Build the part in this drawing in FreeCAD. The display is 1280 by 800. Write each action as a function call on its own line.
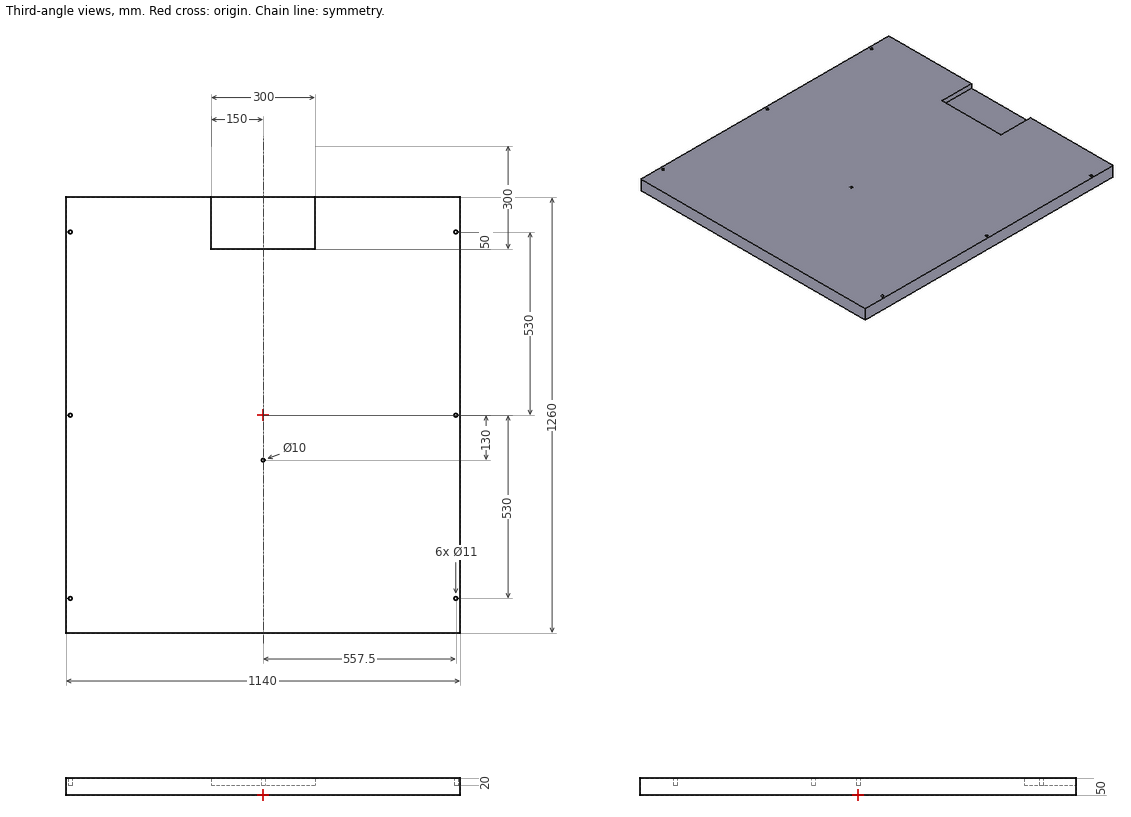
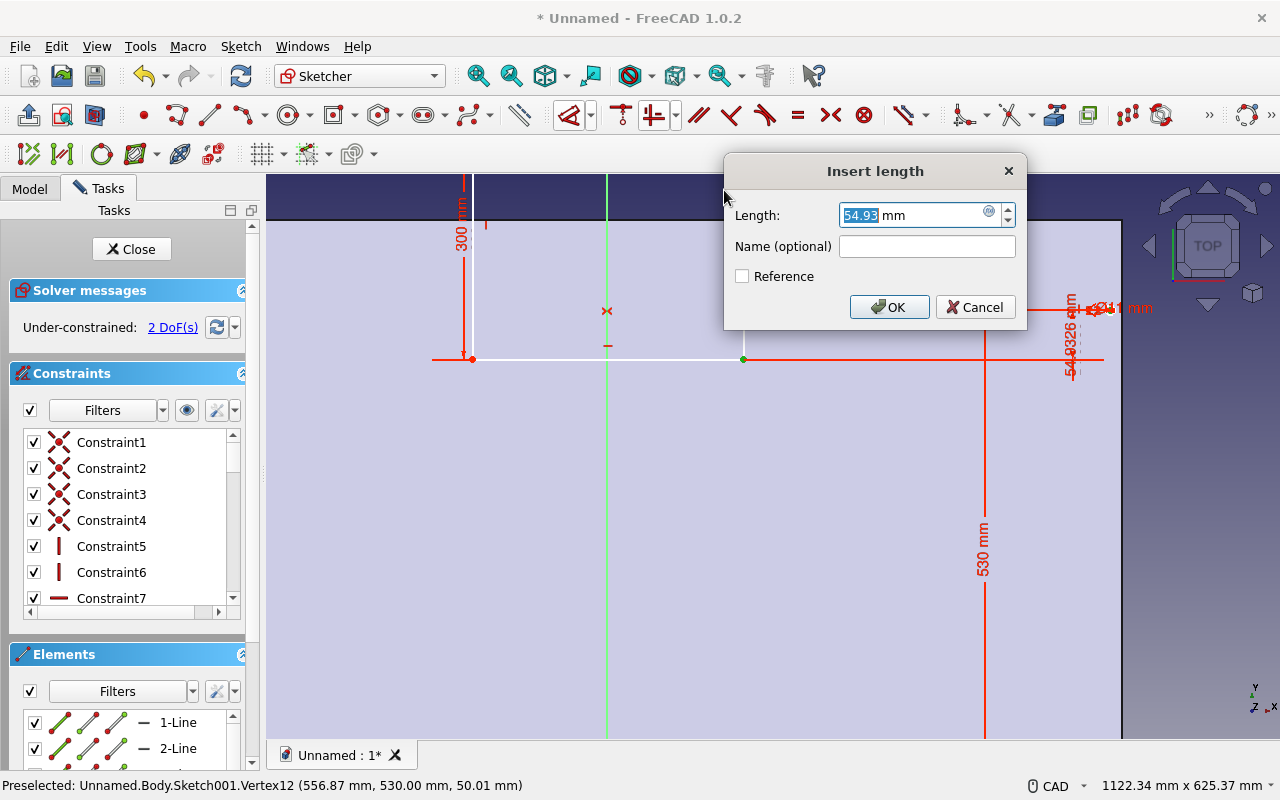
text(50)
key(Return)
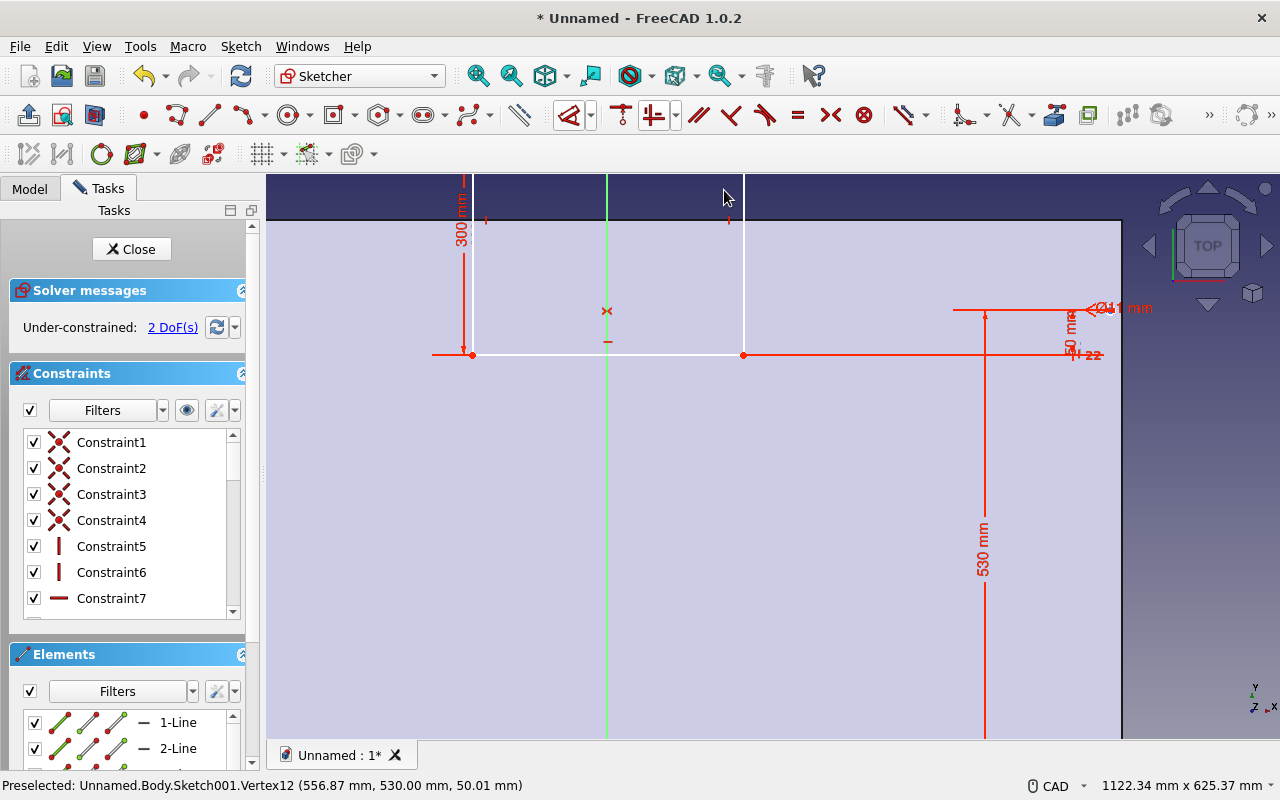
scroll(746, 361, down, 6)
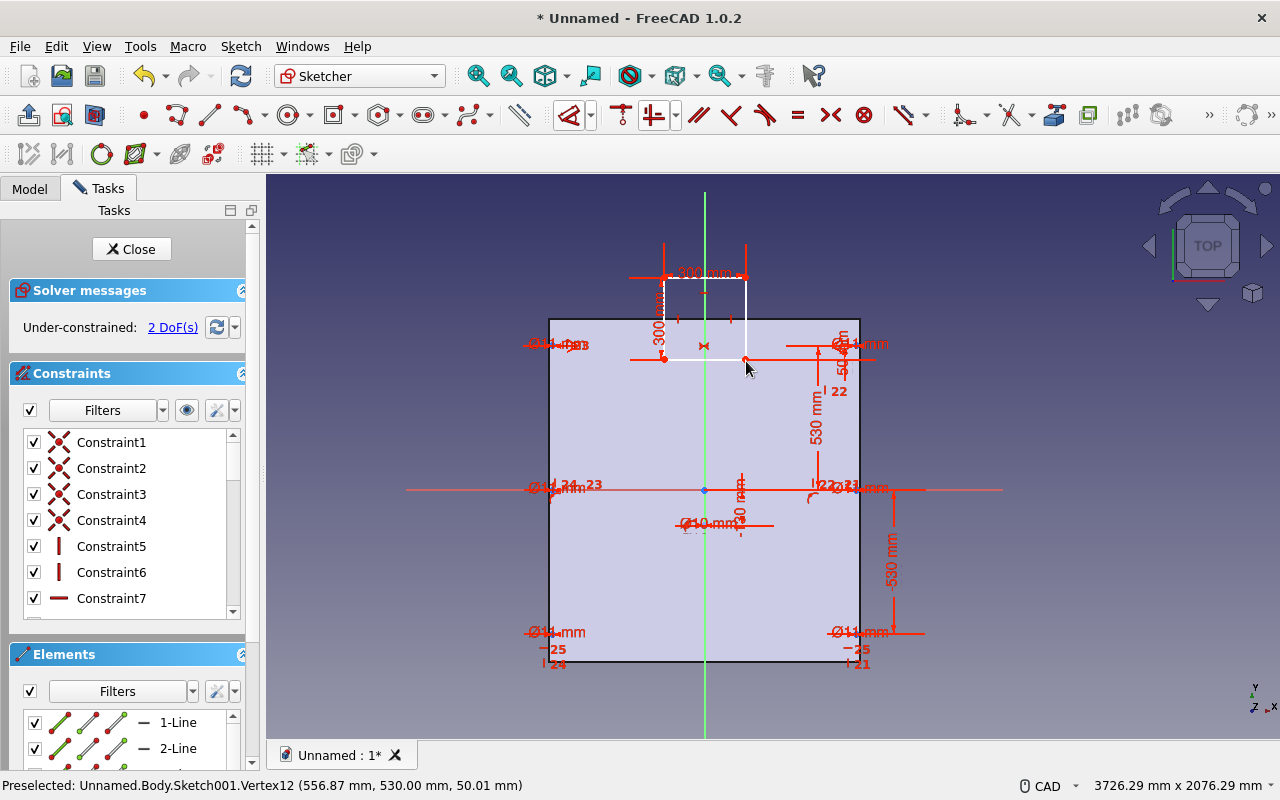
click(664, 278)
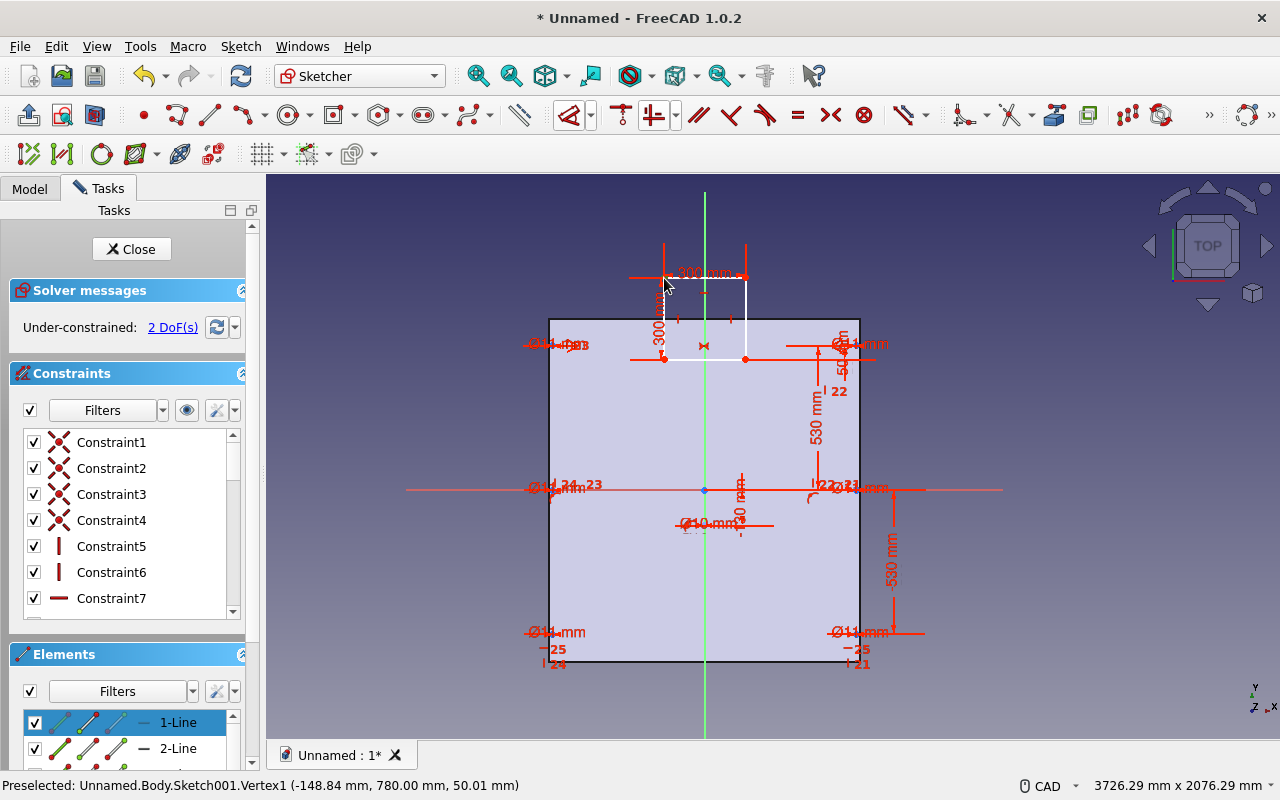
click(590, 116)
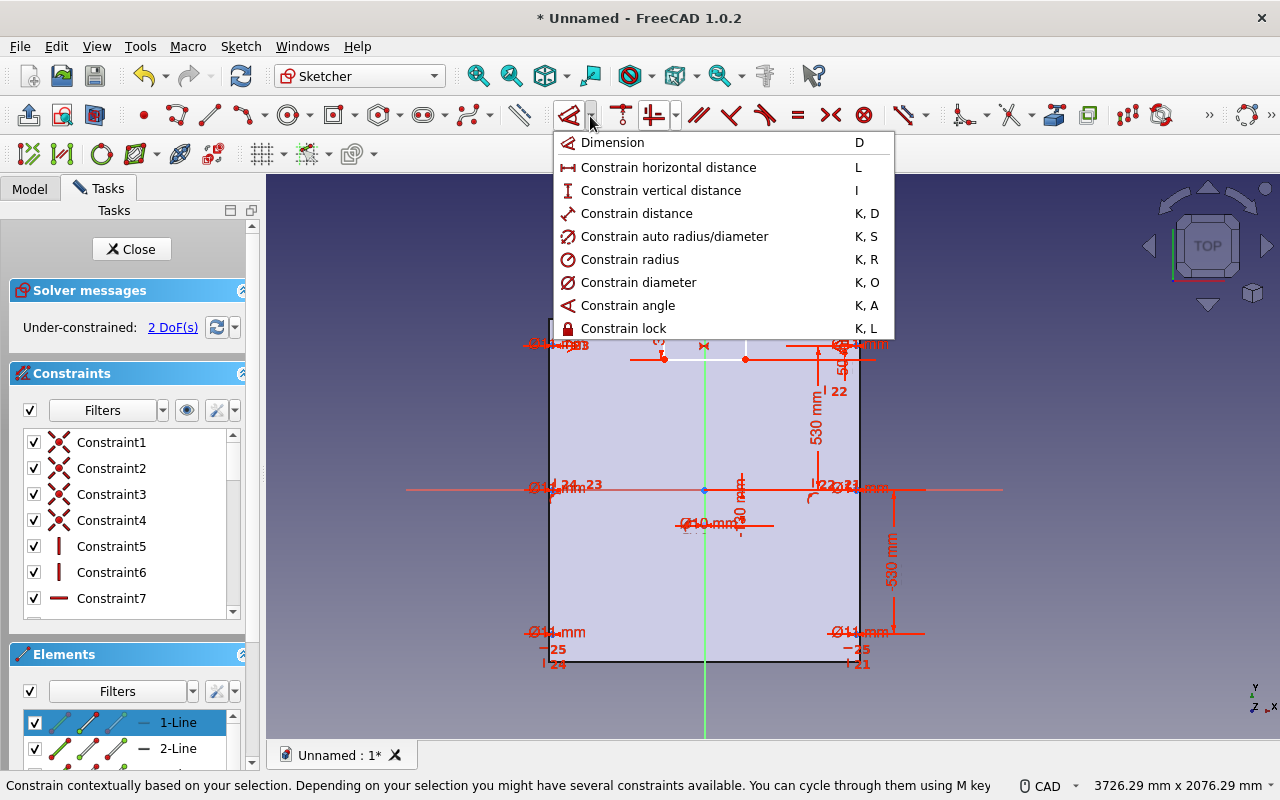
click(724, 168)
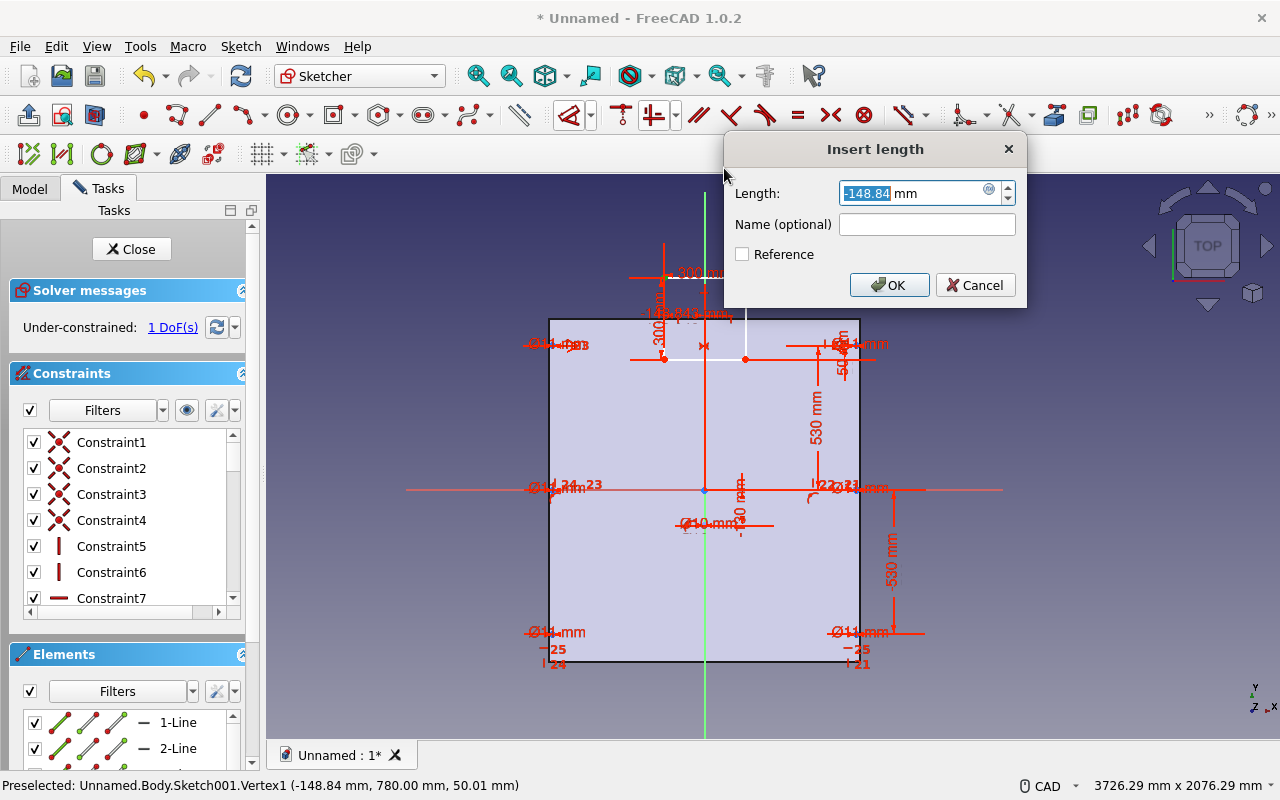
text(-150)
key(Return)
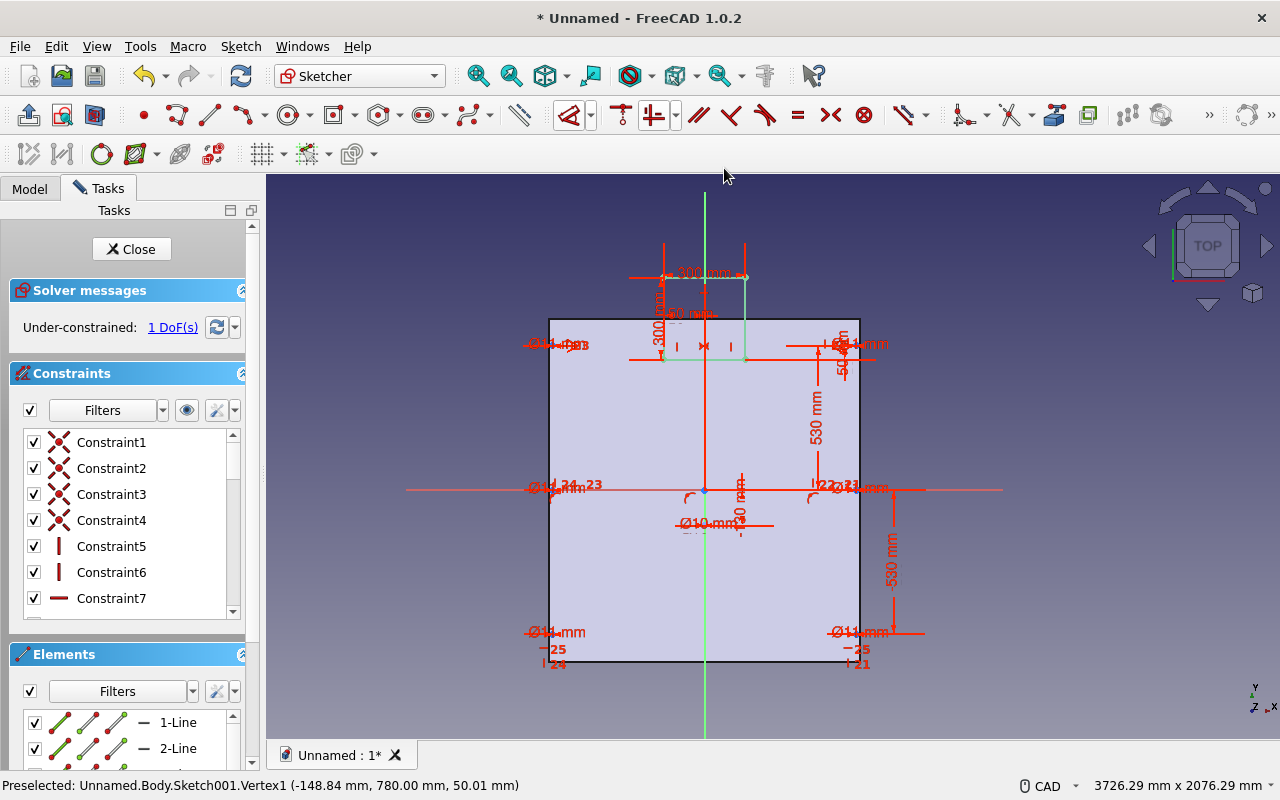
click(856, 634)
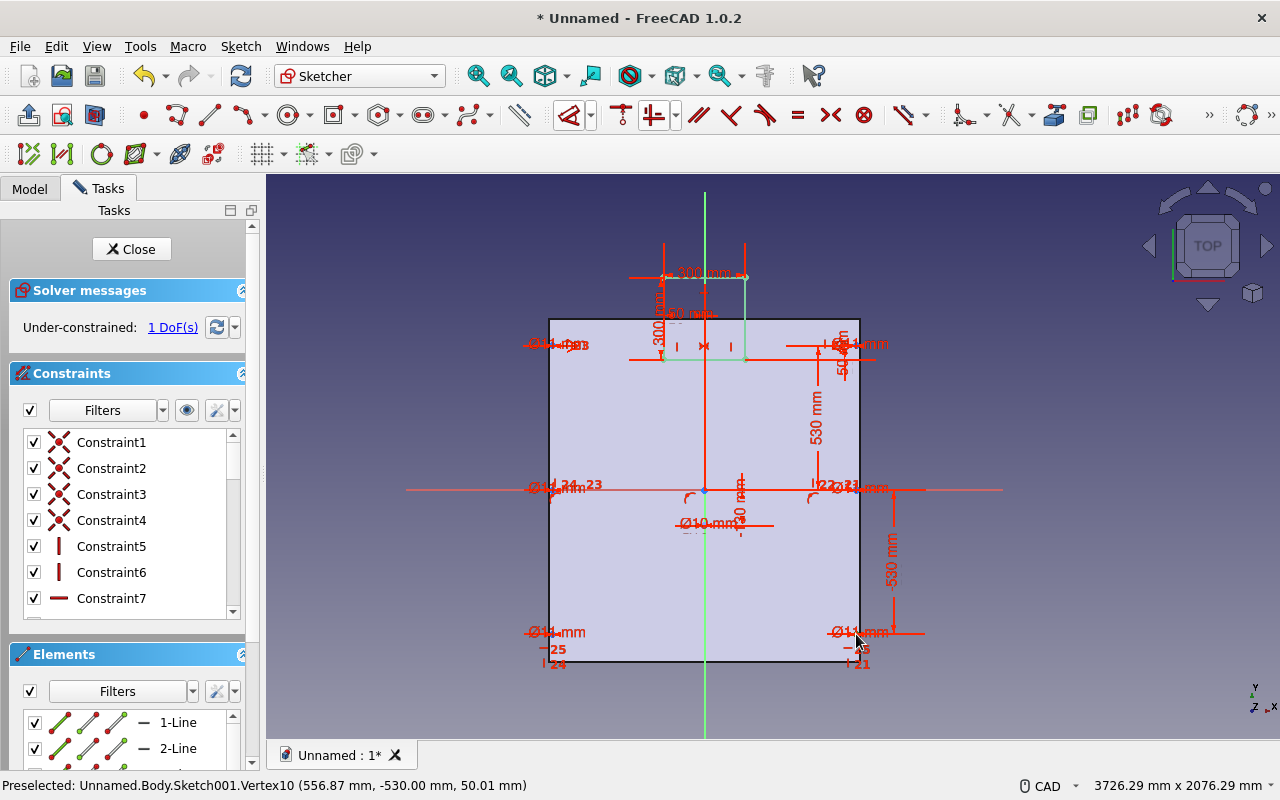
click(590, 116)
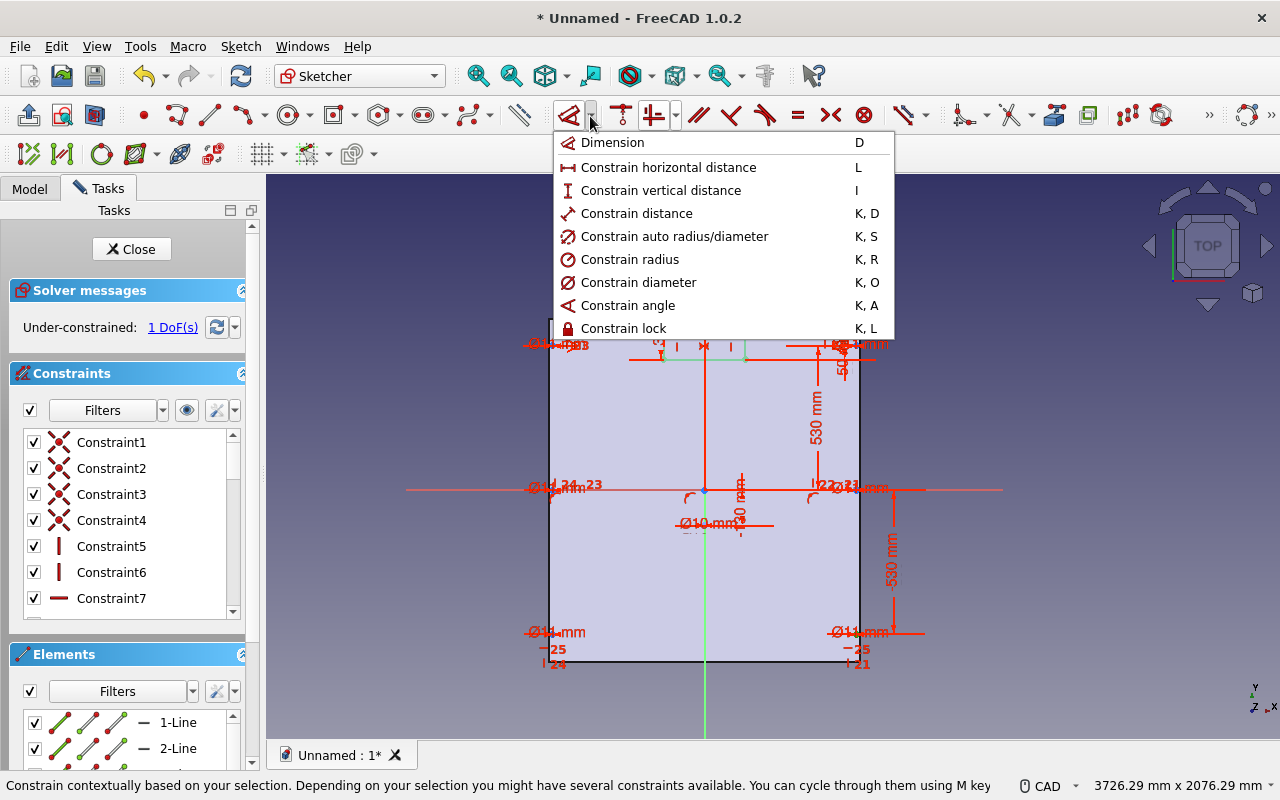
click(724, 168)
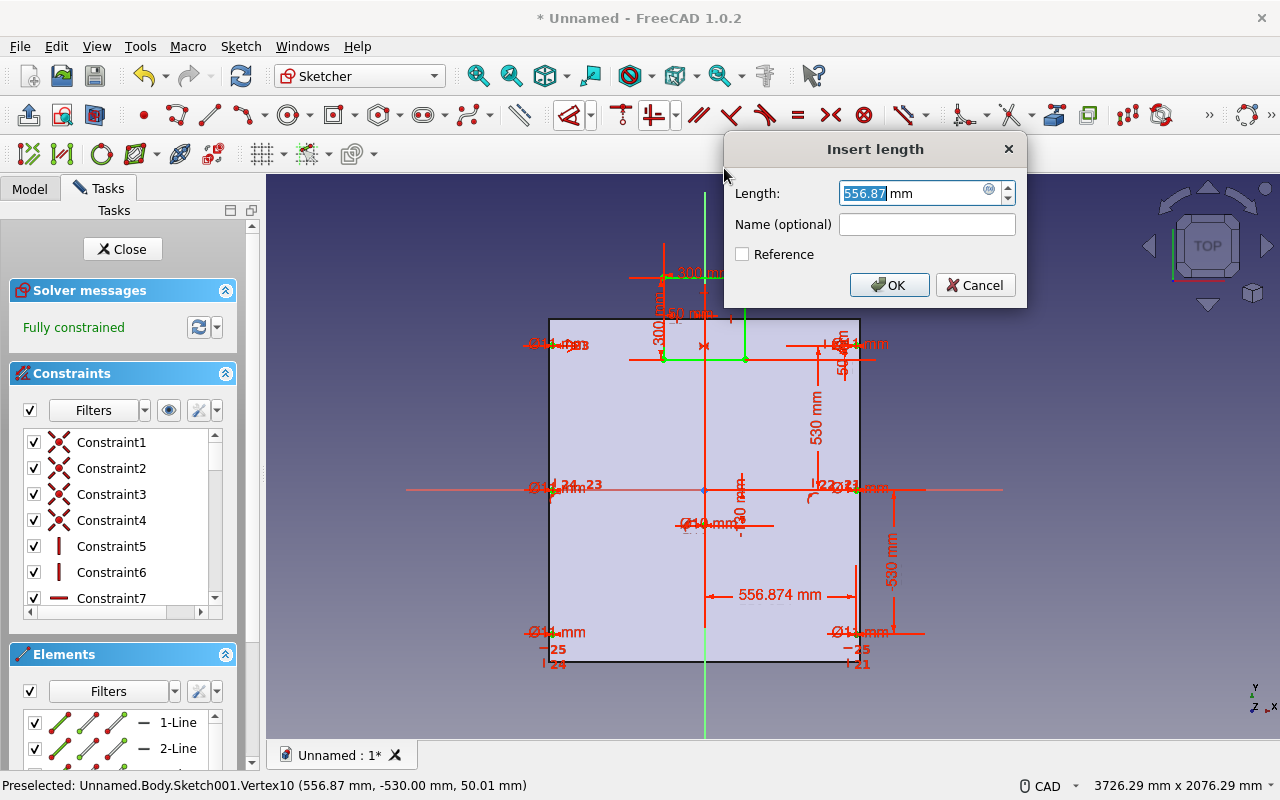
text(557.5)
key(Return)